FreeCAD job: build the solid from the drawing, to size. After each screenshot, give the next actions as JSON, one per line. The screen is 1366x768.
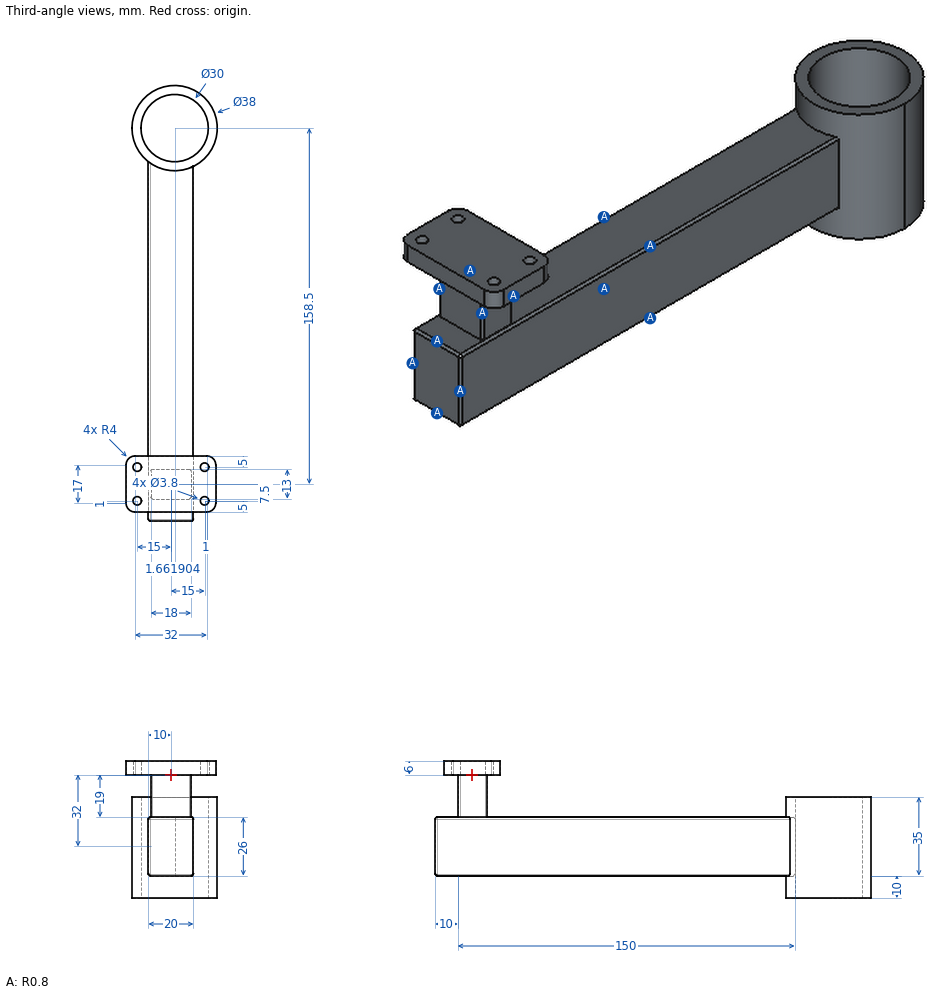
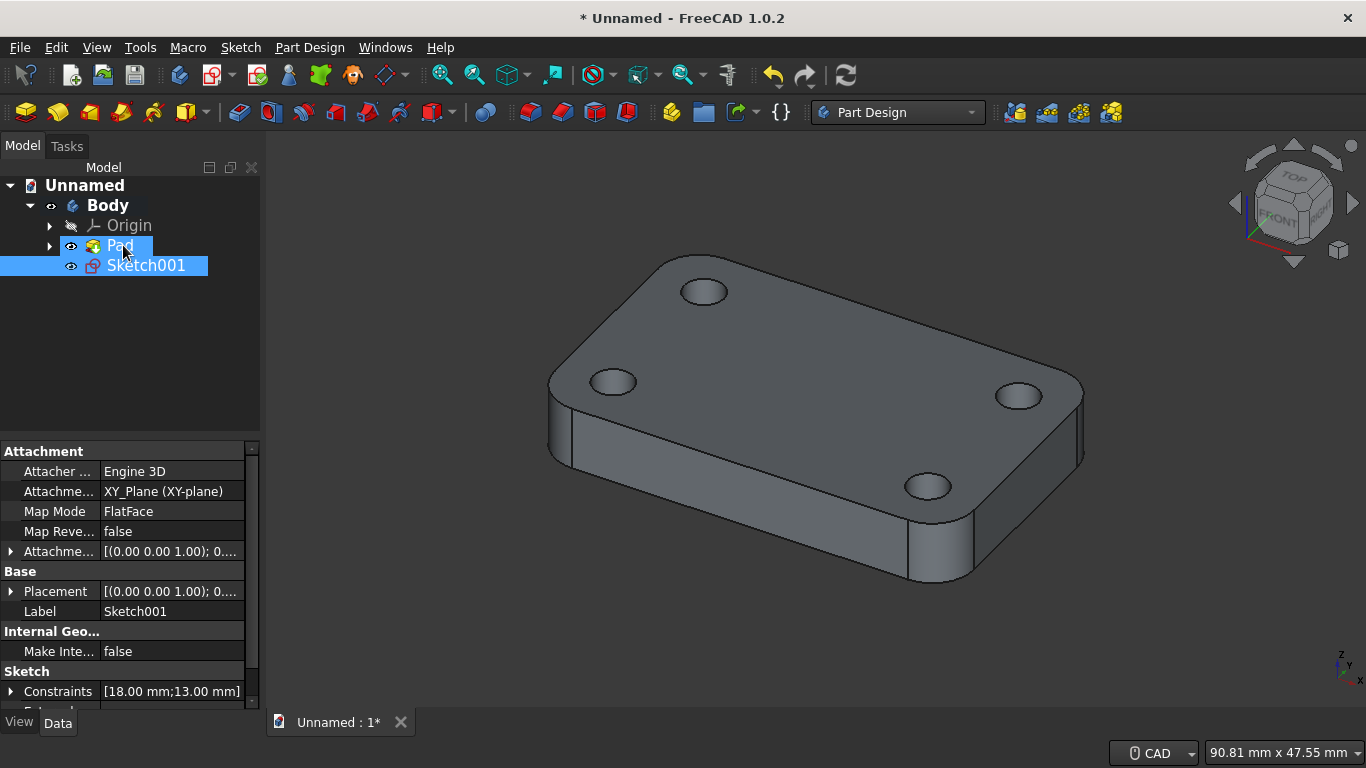
{"action": "left_click", "coordinate": [26, 112]}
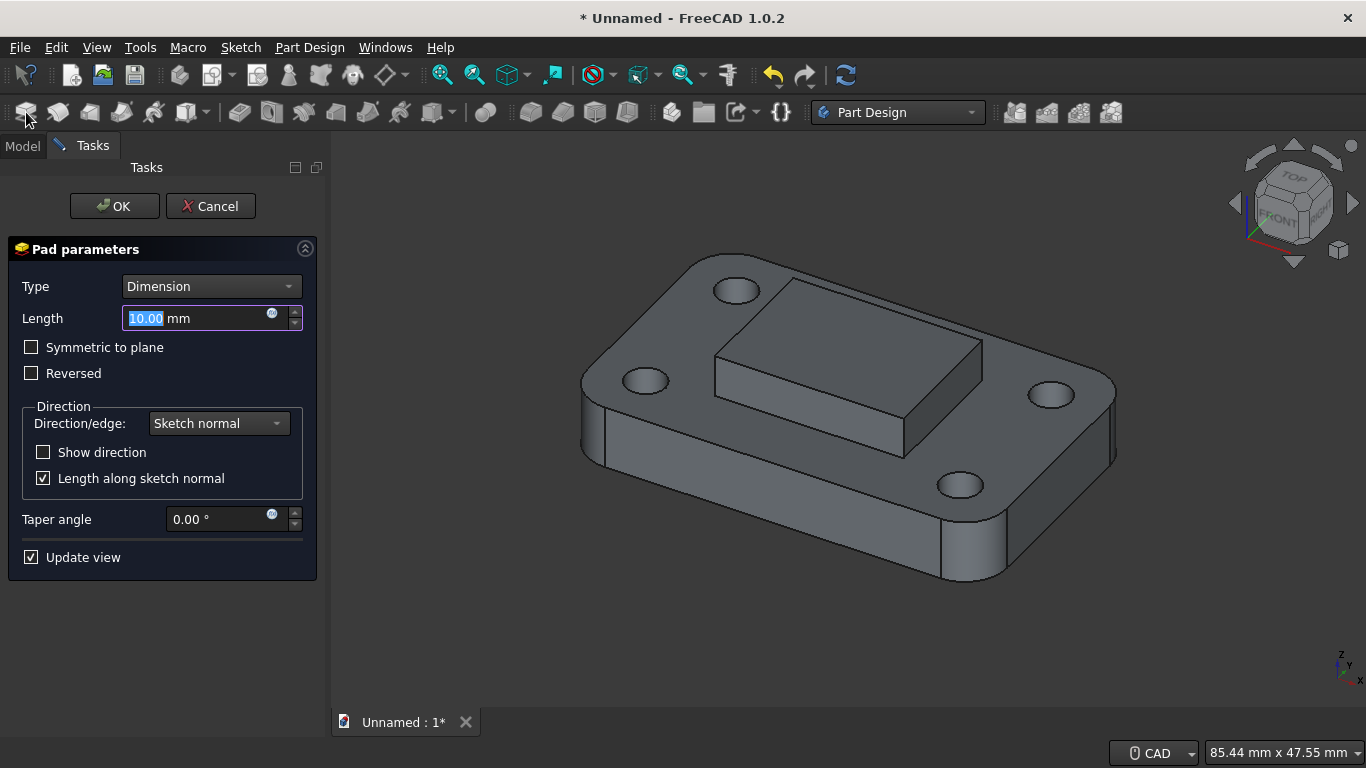
{"action": "type", "text": "32"}
{"action": "key", "text": "Tab"}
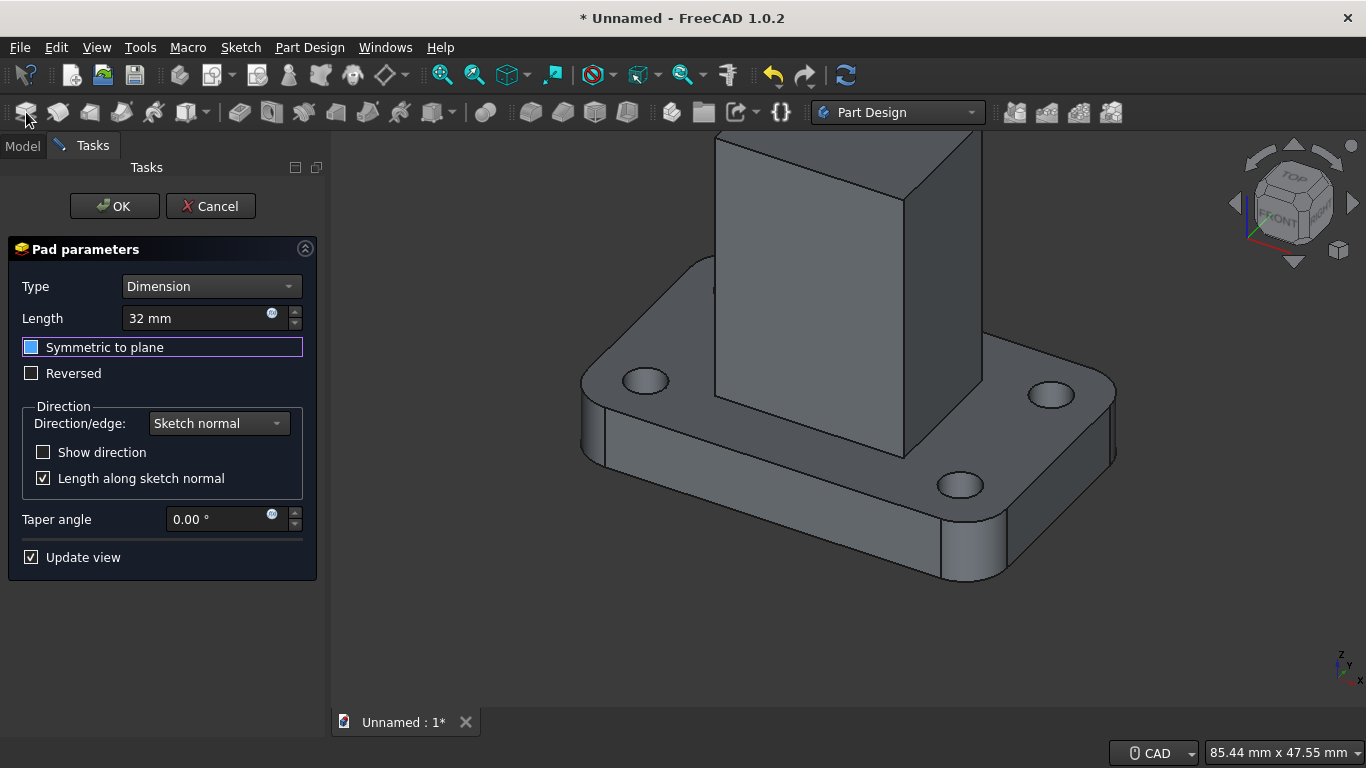
{"action": "left_click", "coordinate": [30, 373]}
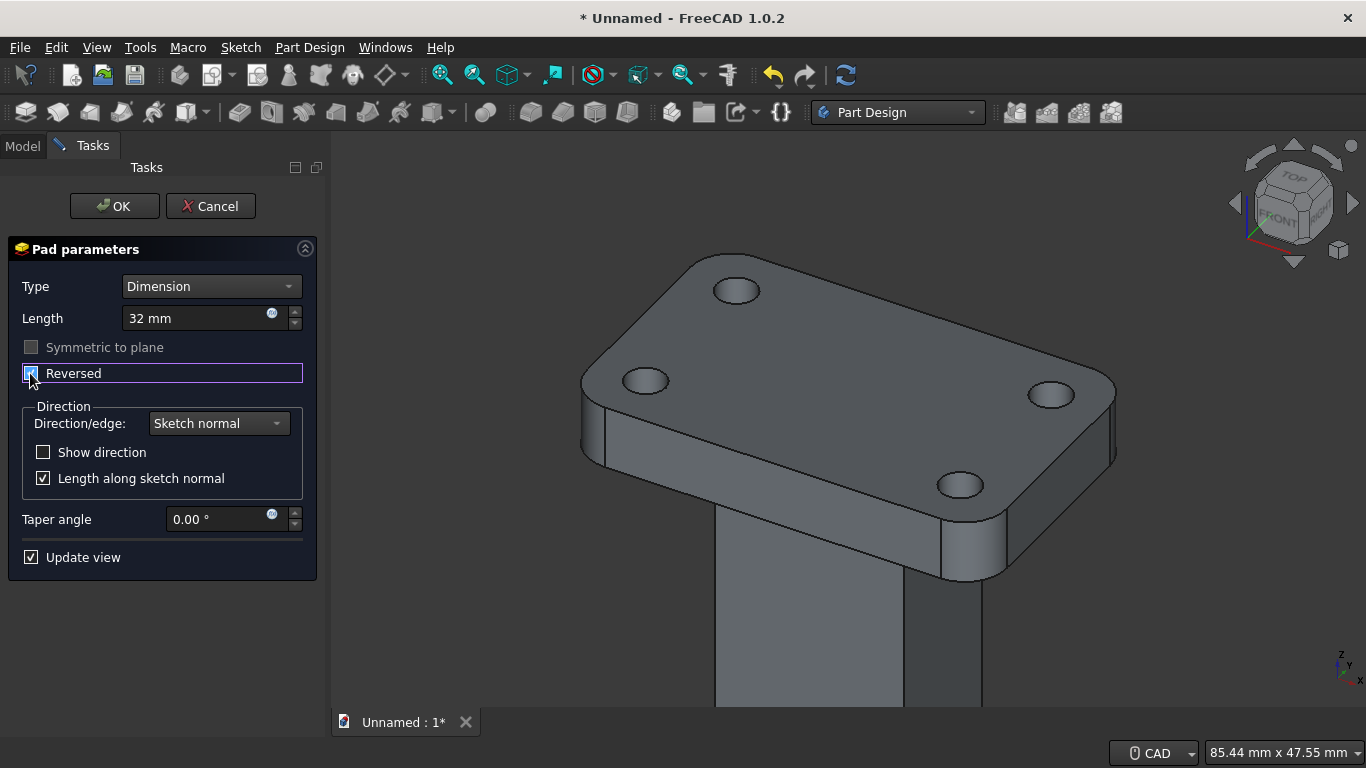
{"action": "left_click", "coordinate": [115, 206]}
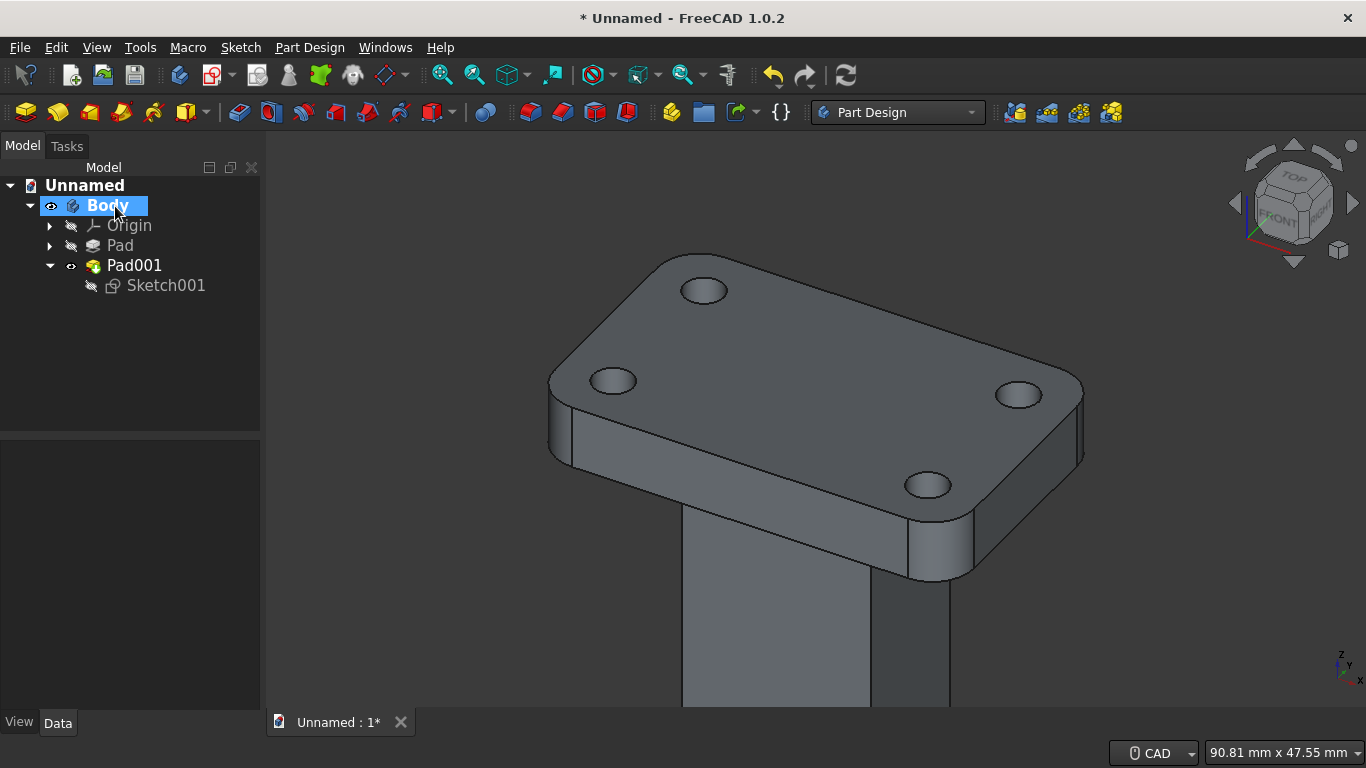
{"action": "left_click", "coordinate": [444, 76]}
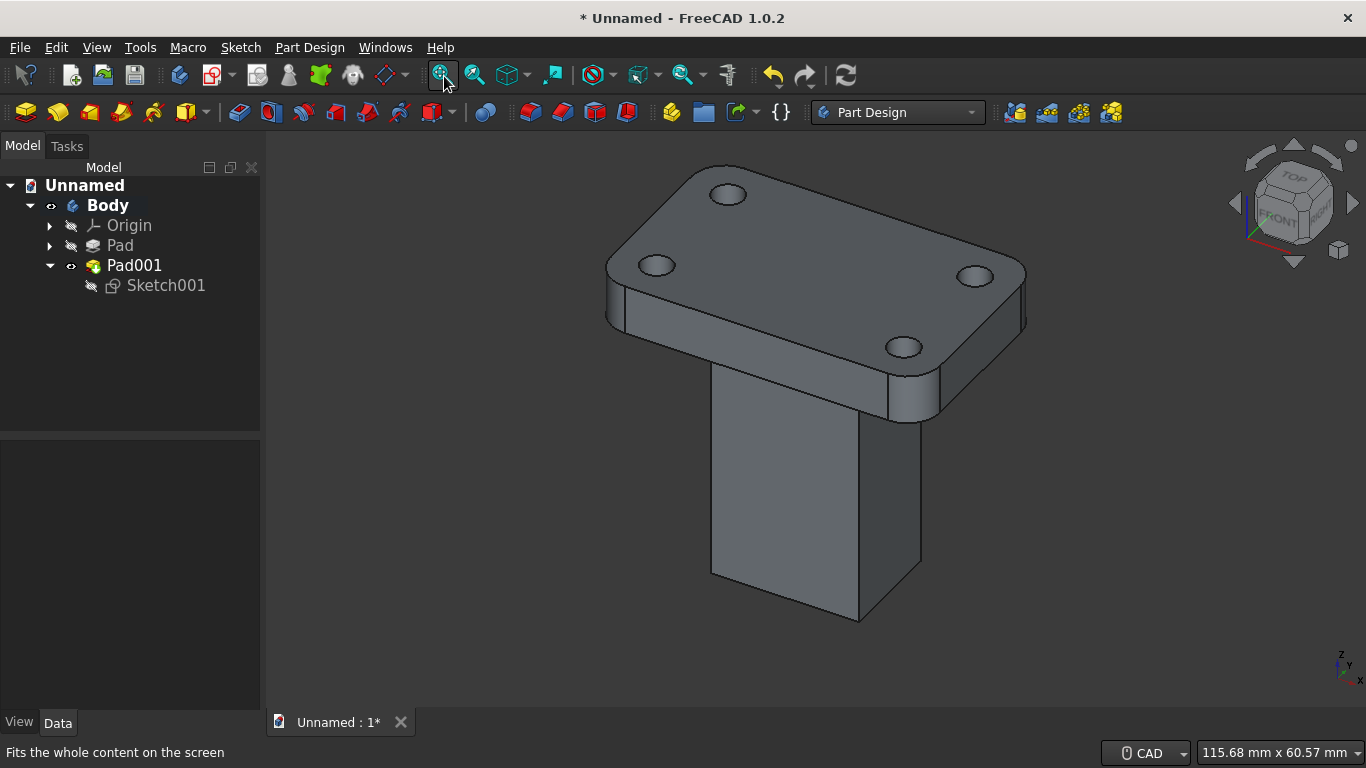
{"action": "left_click", "coordinate": [785, 436]}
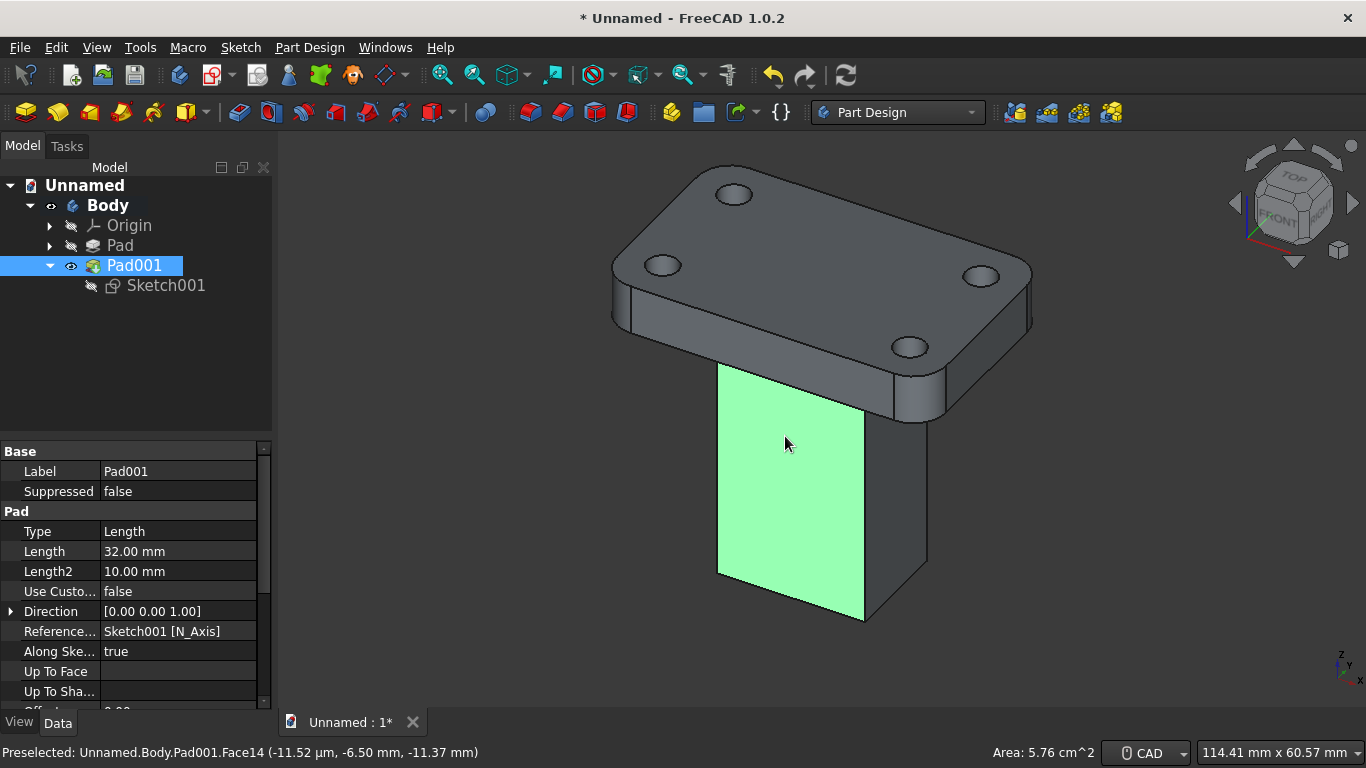
{"action": "left_click", "coordinate": [212, 76]}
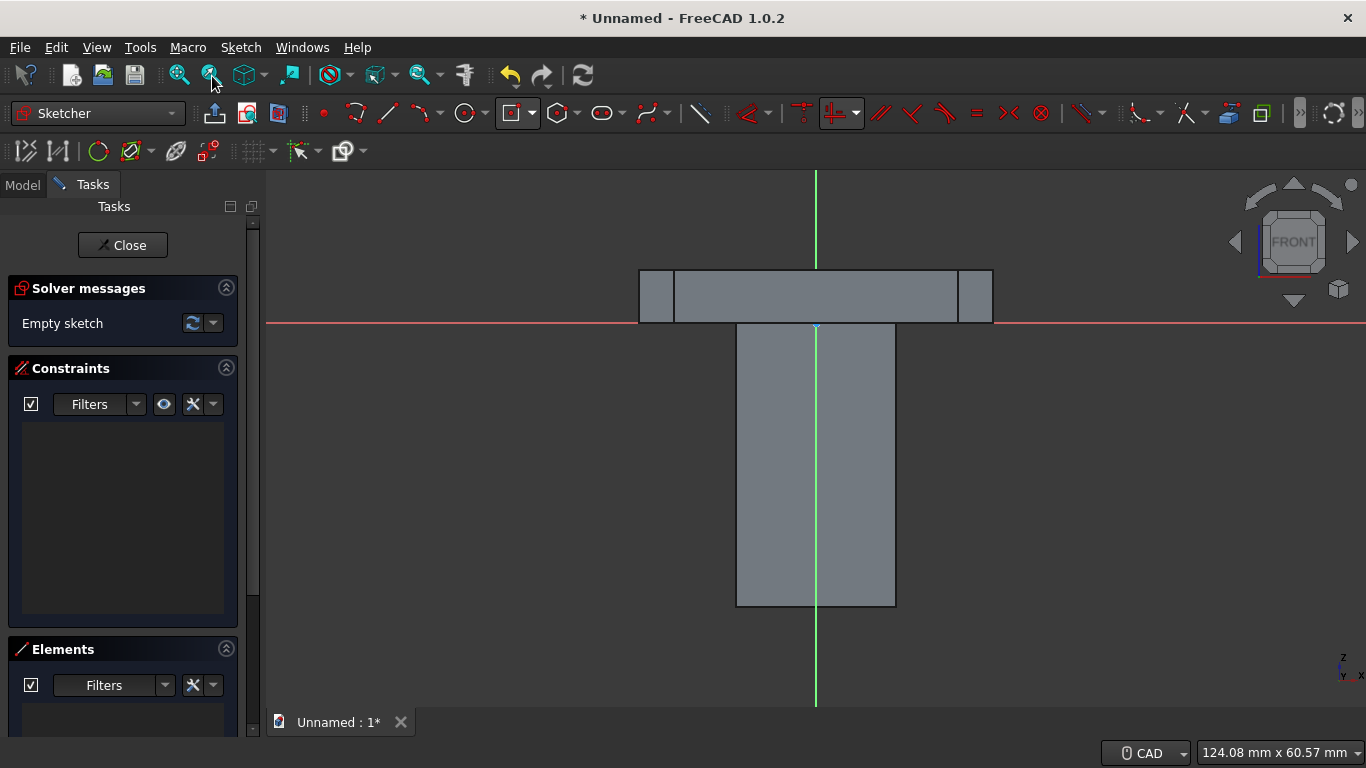
{"action": "scroll", "coordinate": [438, 198], "scroll_direction": "down", "scroll_amount": 1}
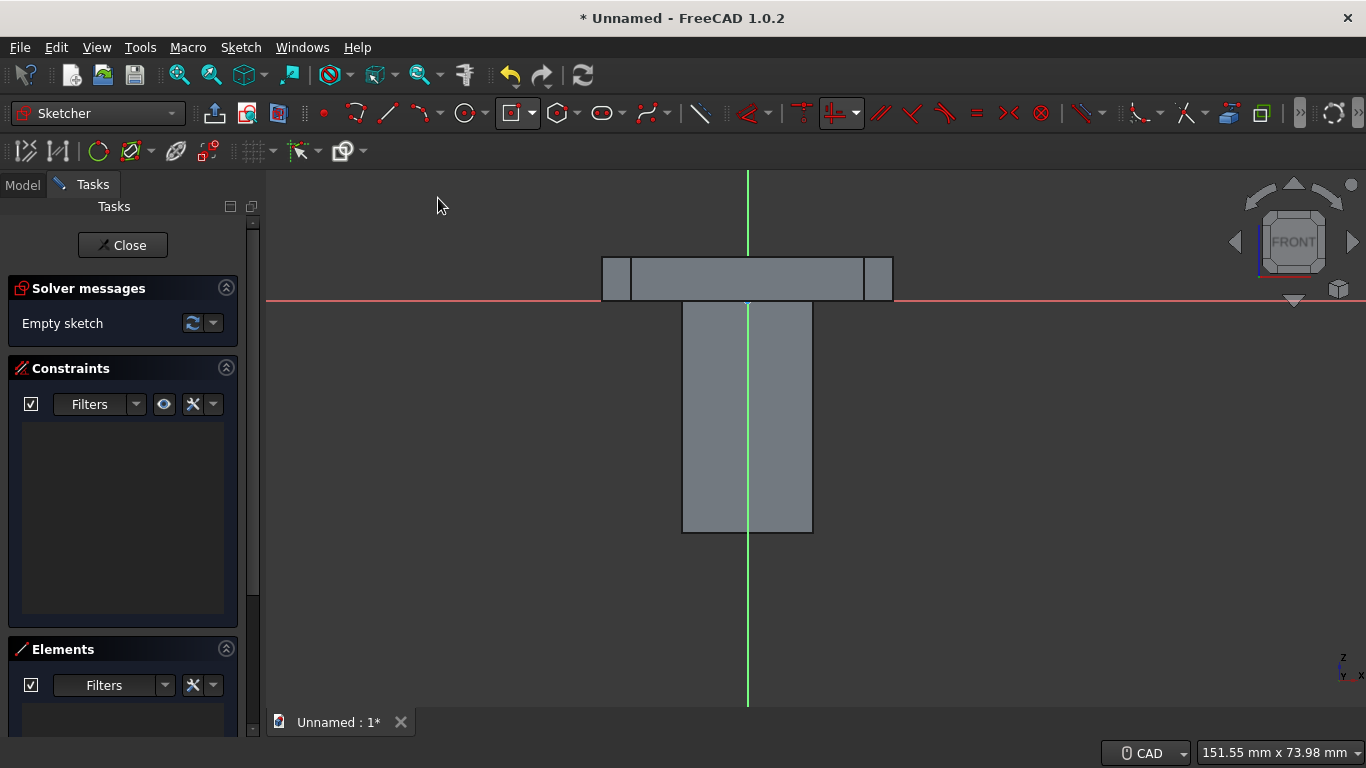
{"action": "key", "text": "g r"}